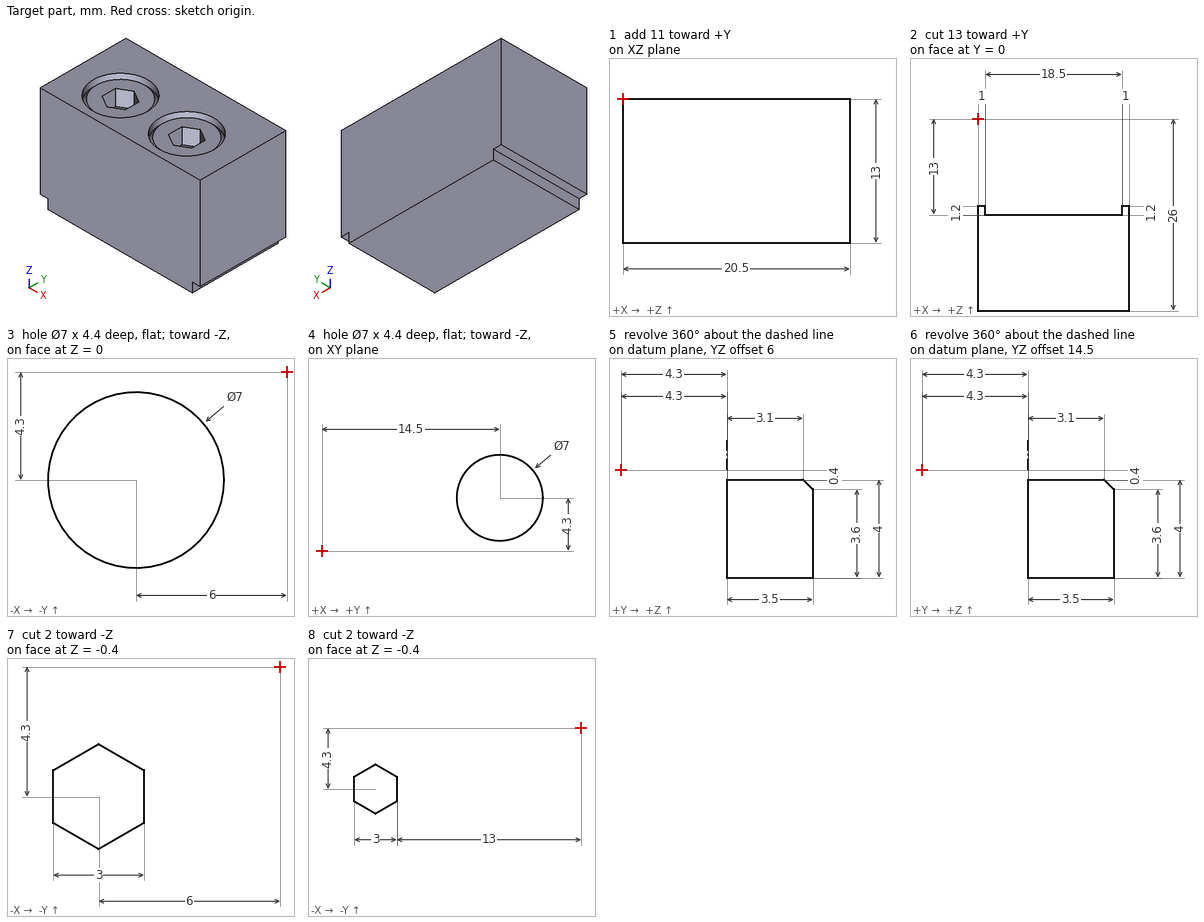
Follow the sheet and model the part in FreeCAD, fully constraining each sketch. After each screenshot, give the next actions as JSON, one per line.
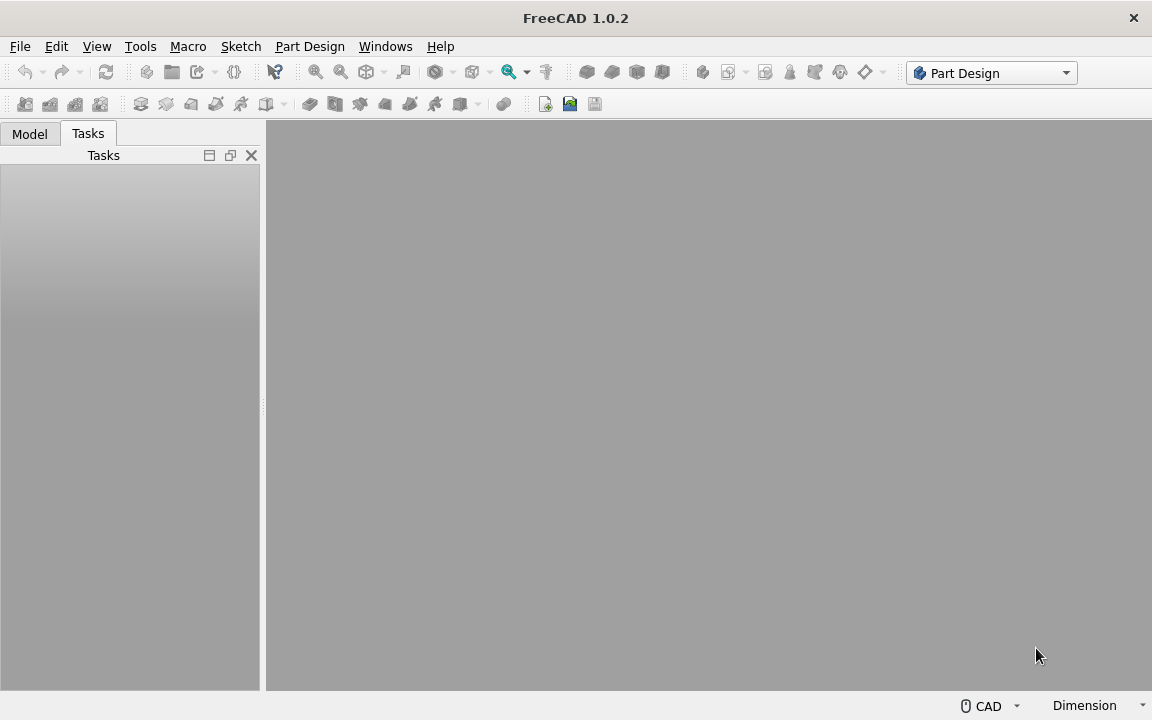
{"action": "key", "text": "ctrl+n"}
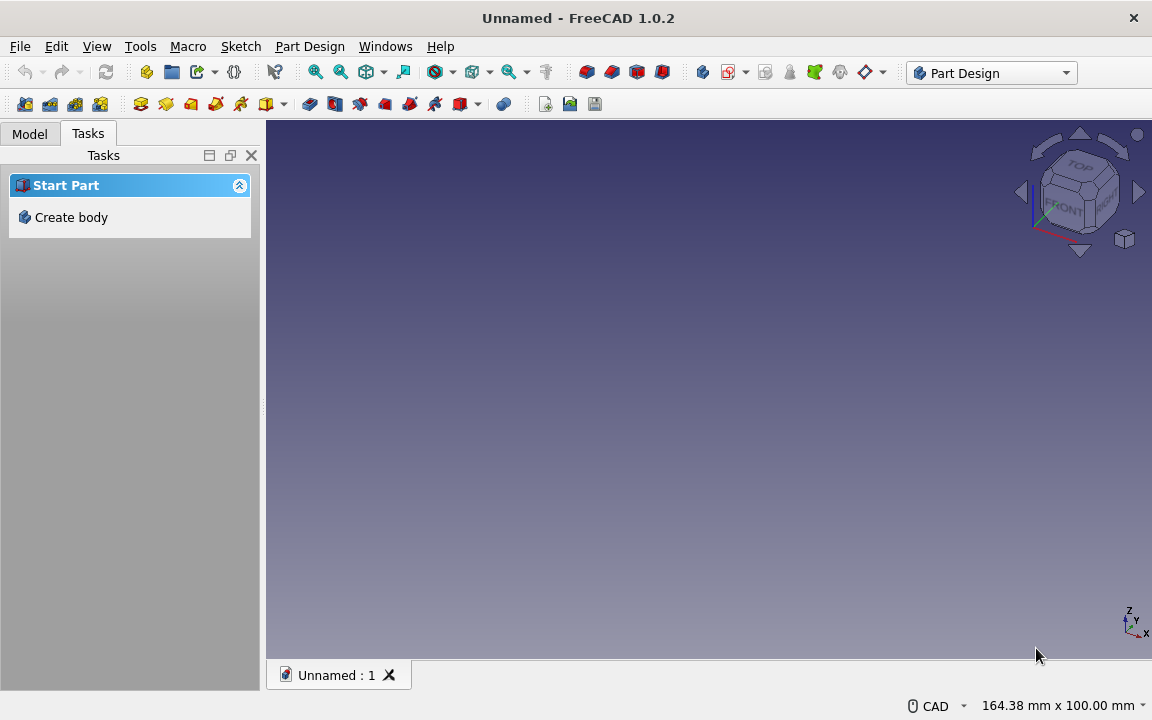
{"action": "left_click", "coordinate": [728, 72]}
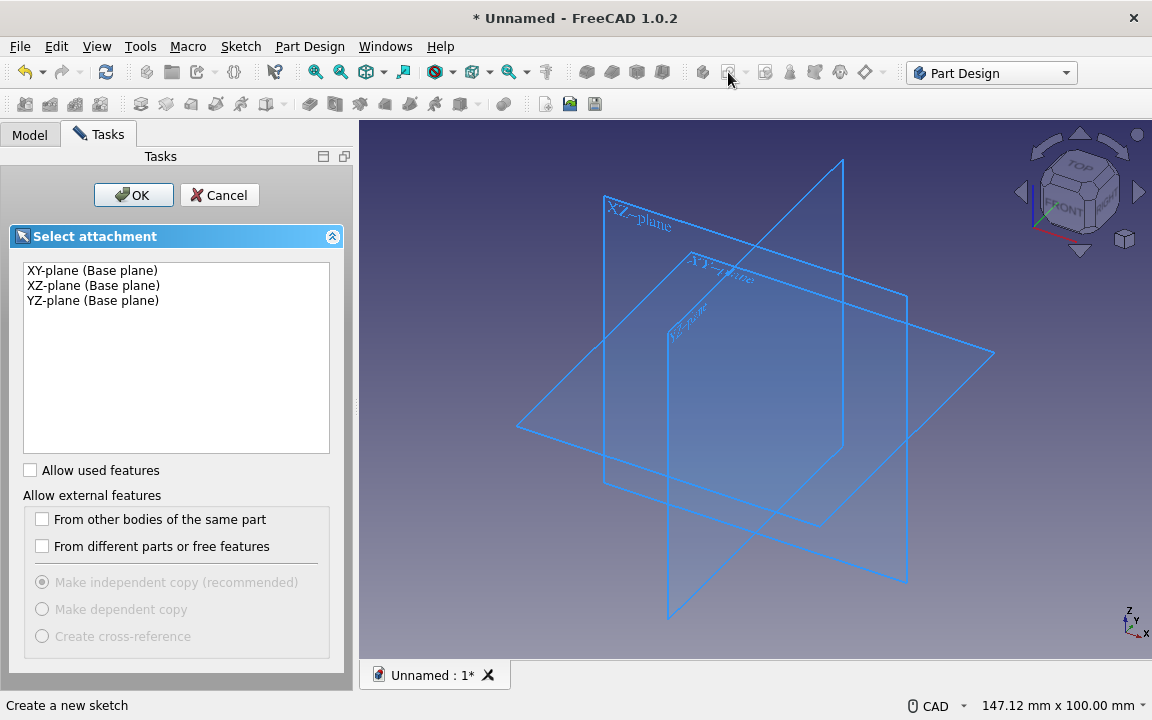
{"action": "left_click", "coordinate": [84, 286]}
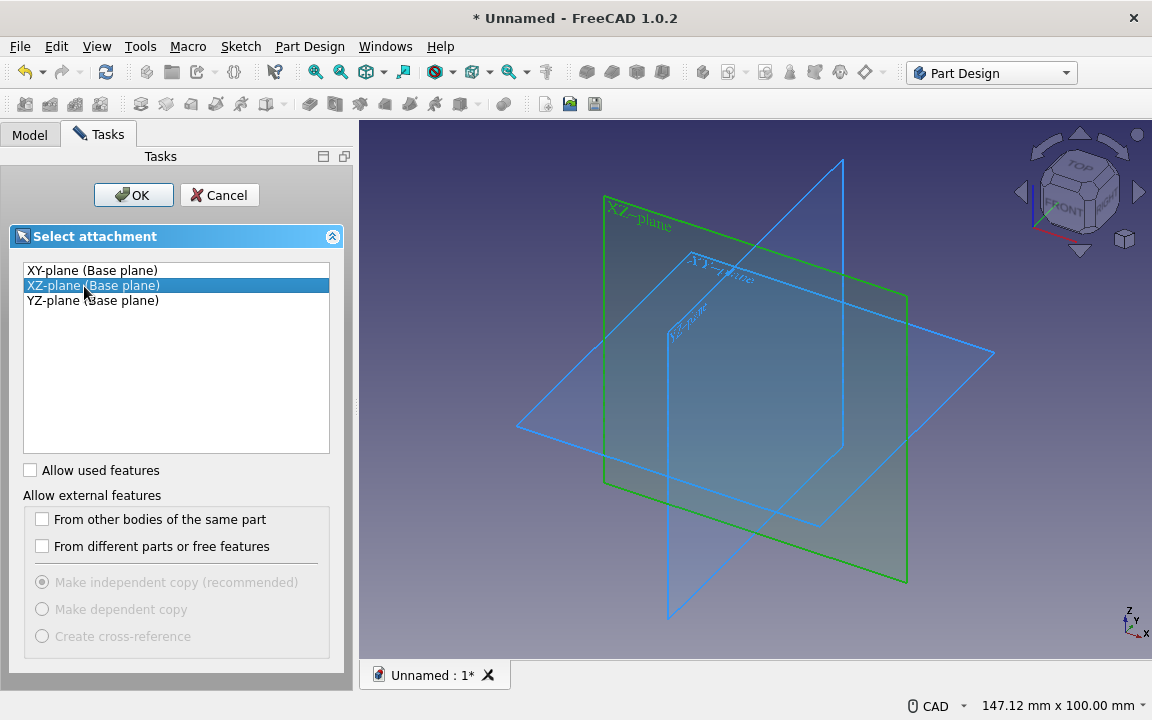
{"action": "left_click", "coordinate": [134, 195]}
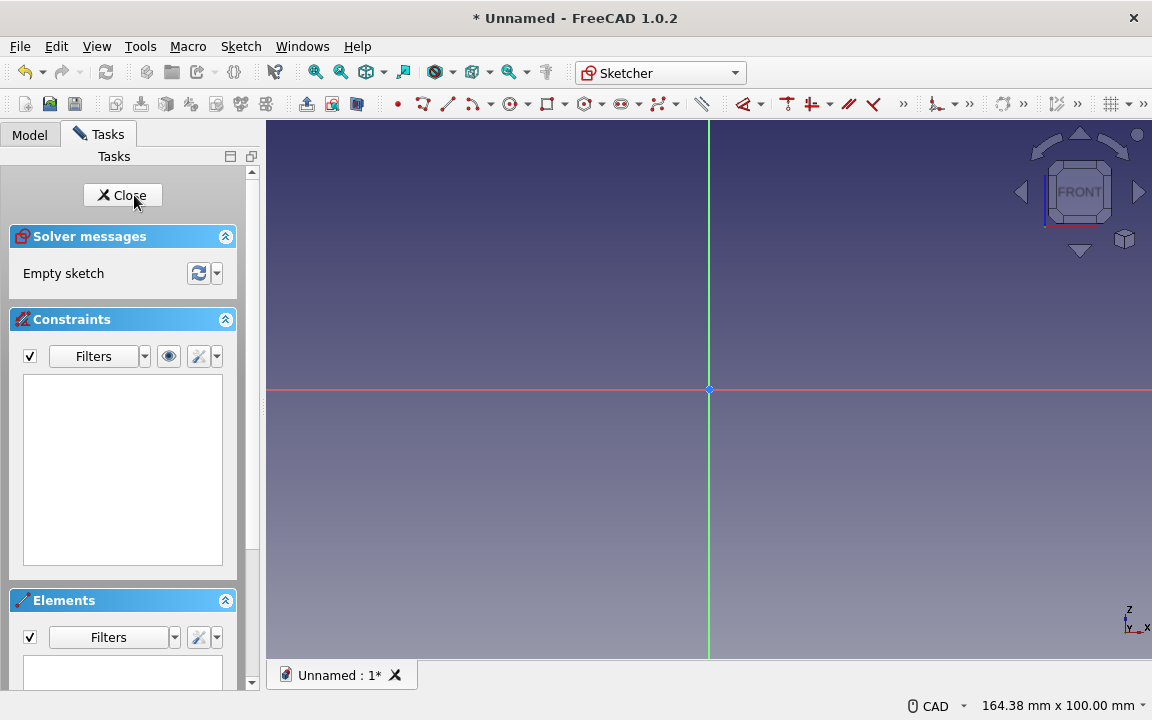
{"action": "scroll", "coordinate": [805, 436], "scroll_direction": "up", "scroll_amount": 7}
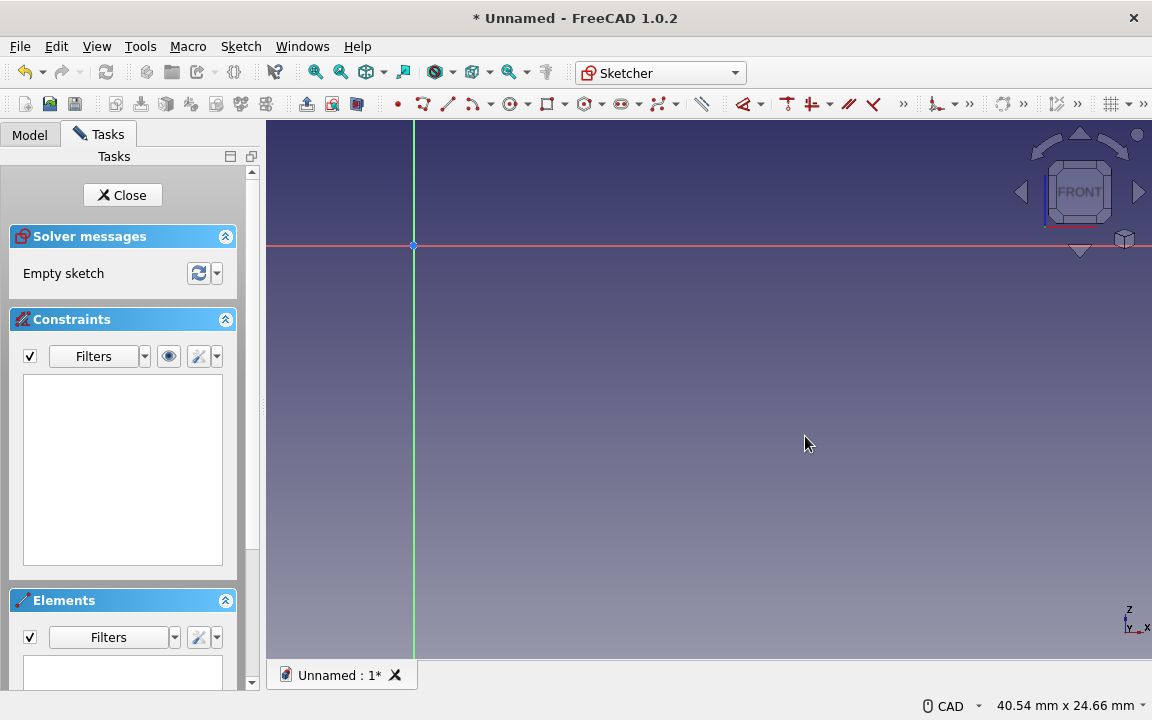
{"action": "left_click", "coordinate": [546, 104]}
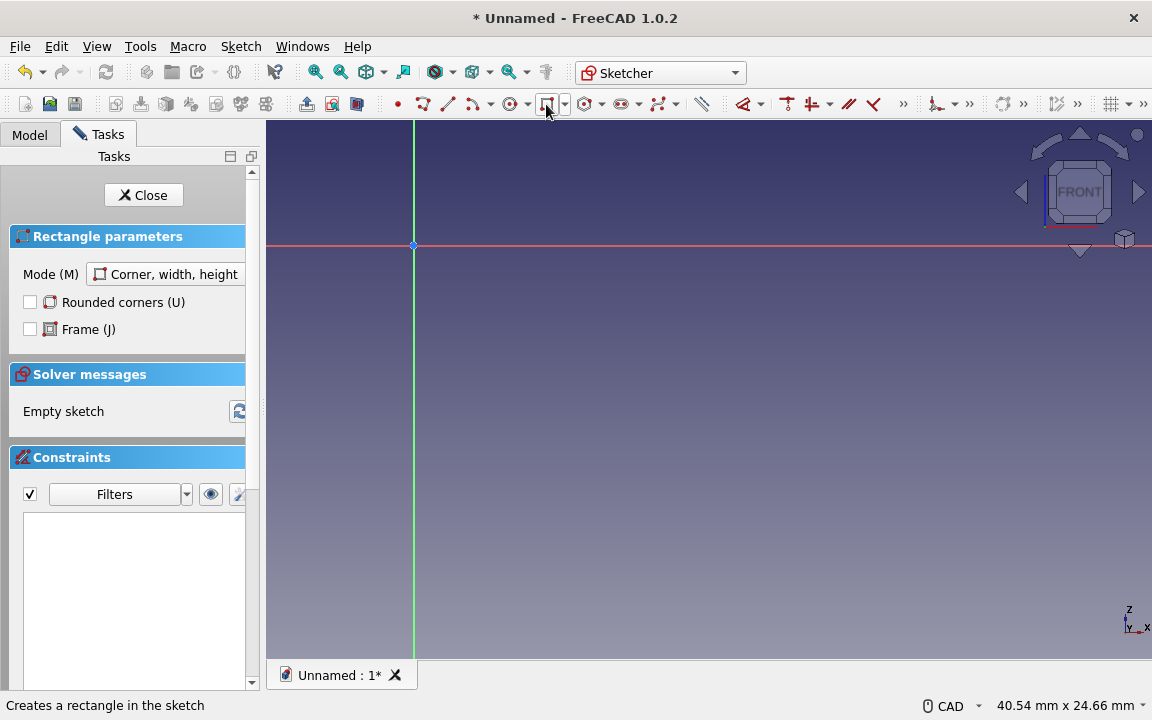
{"action": "left_click", "coordinate": [414, 246]}
{"action": "mouse_move", "coordinate": [862, 530]}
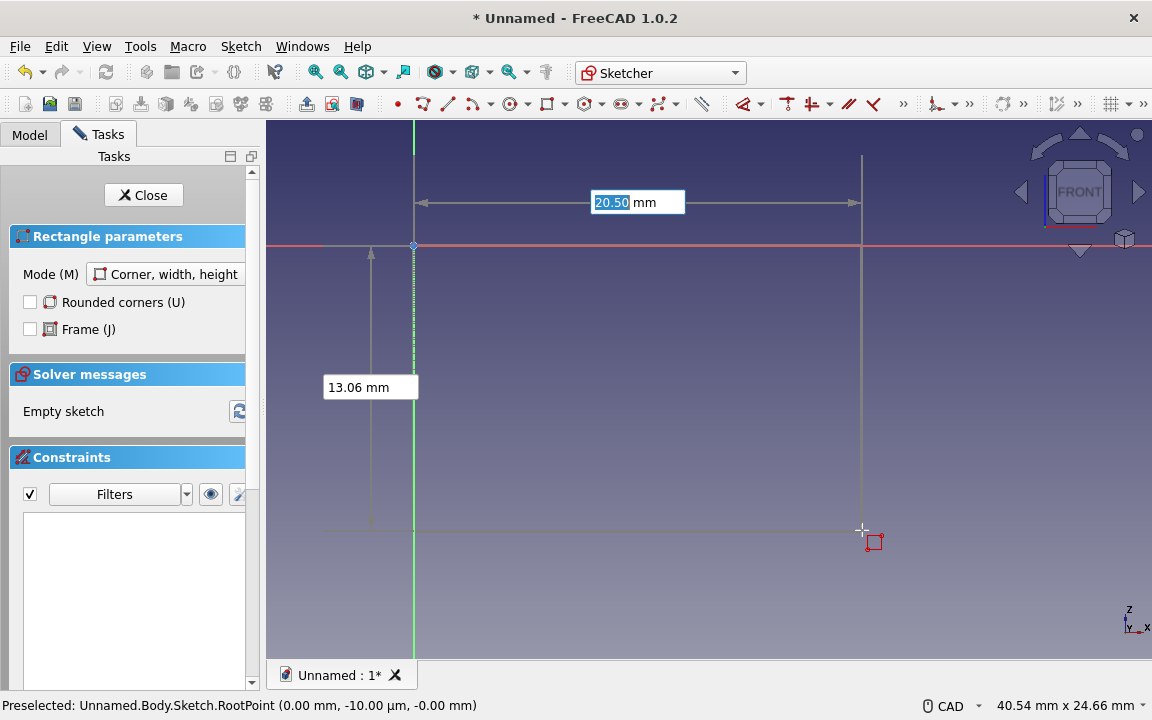
{"action": "type", "text": "20.5"}
{"action": "key", "text": "Tab"}
{"action": "type", "text": "13"}
{"action": "key", "text": "Return"}
{"action": "key", "text": "Escape"}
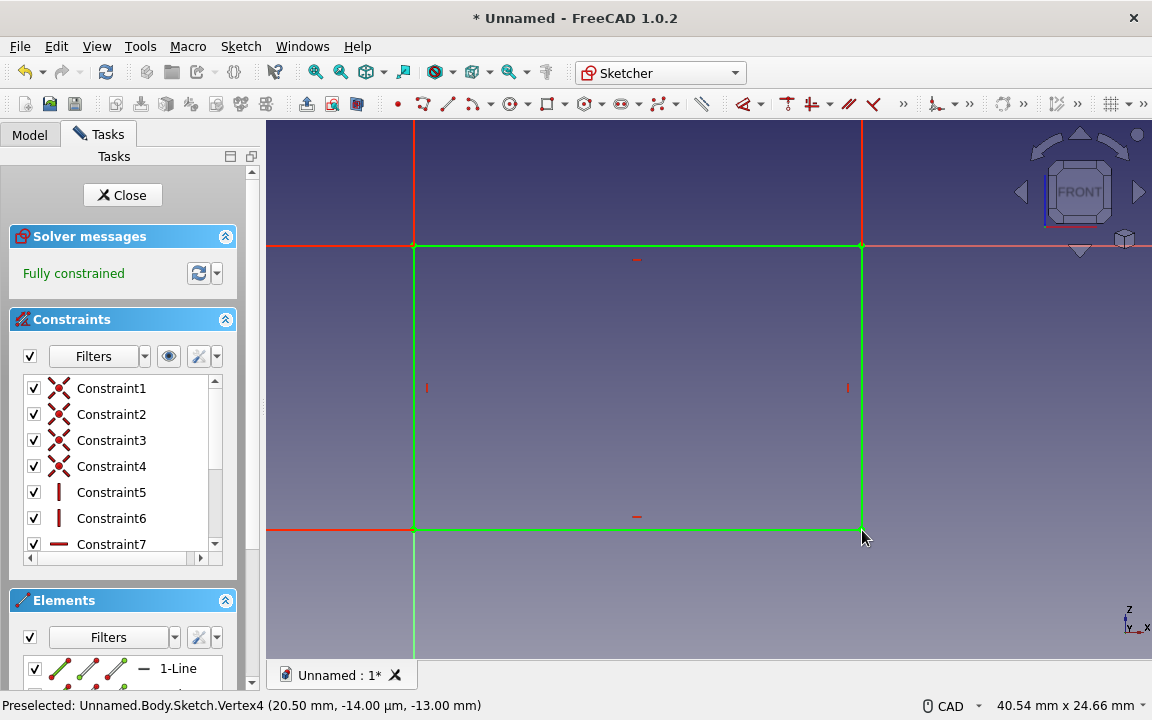
{"action": "left_click", "coordinate": [123, 195]}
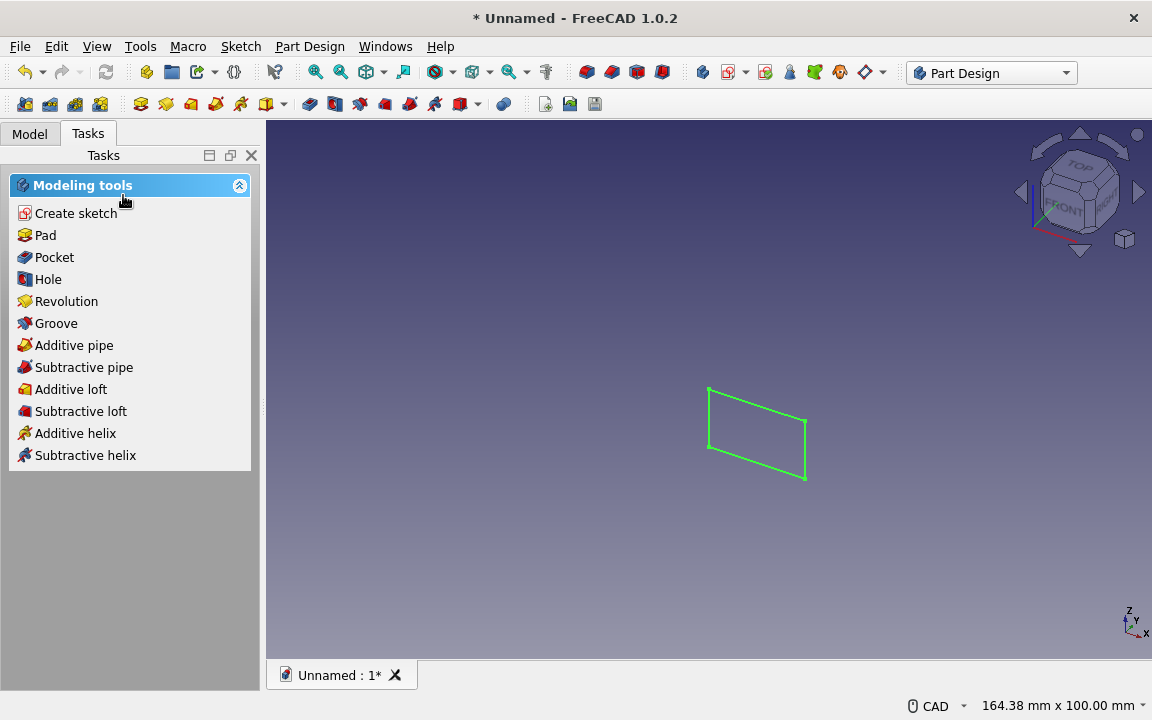
{"action": "left_click", "coordinate": [141, 104]}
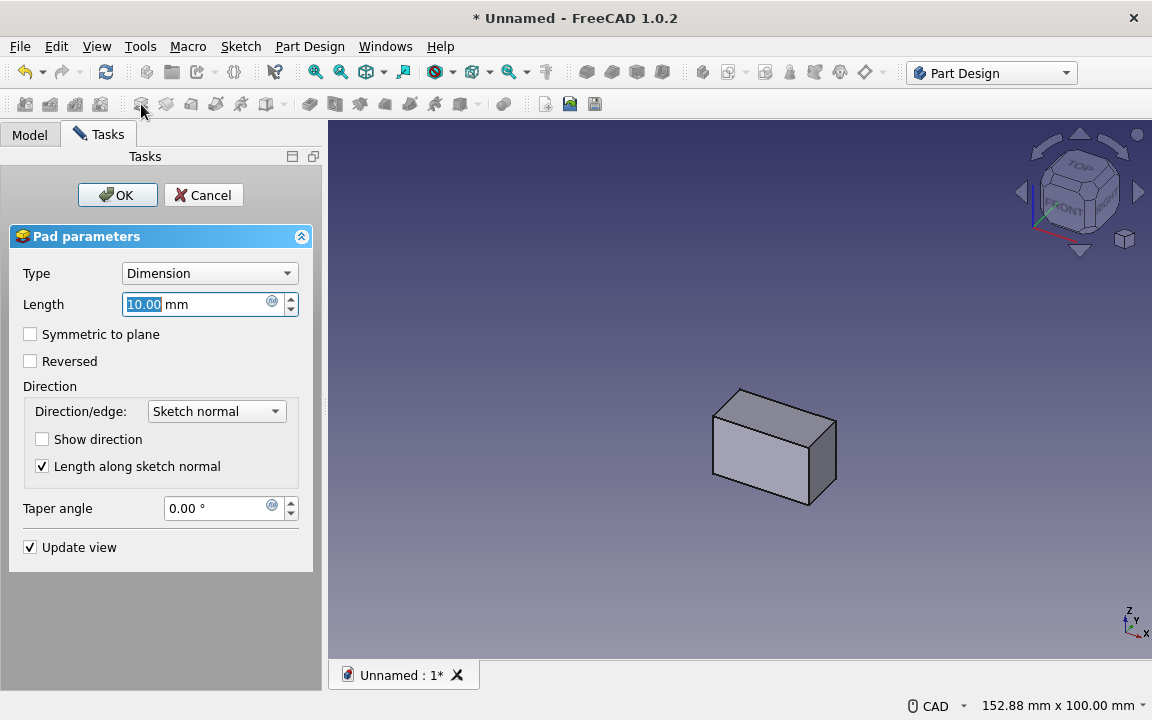
{"action": "type", "text": "11"}
{"action": "key", "text": "Tab"}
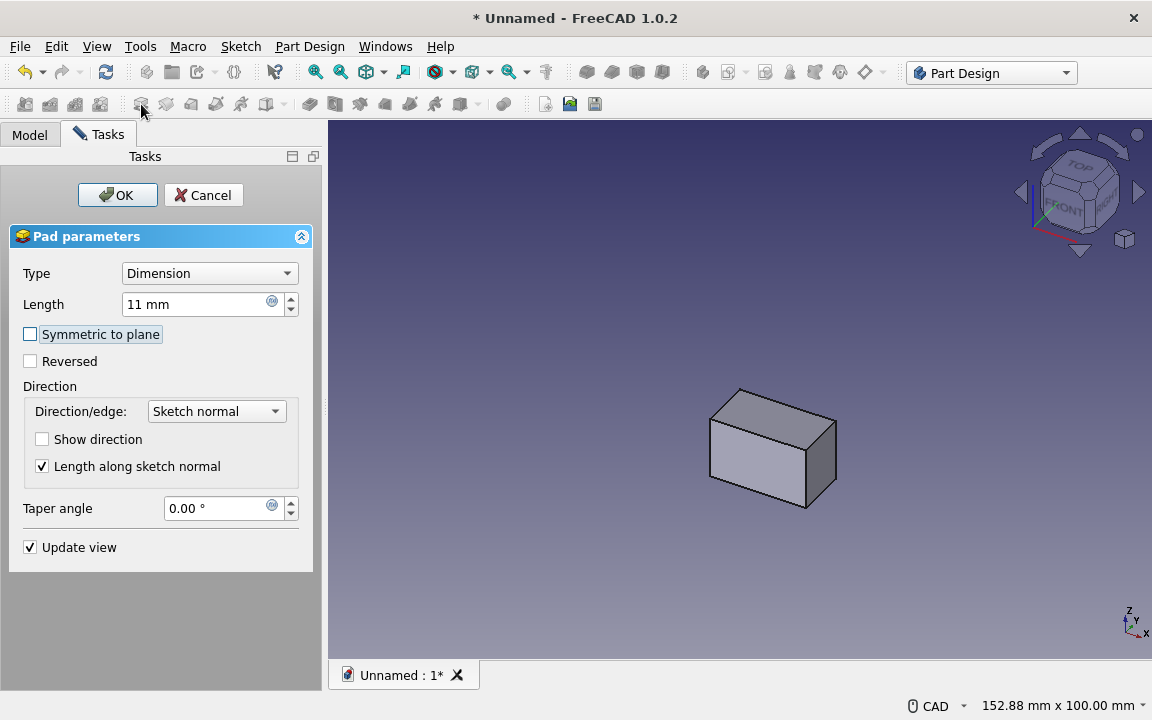
{"action": "left_click", "coordinate": [31, 361]}